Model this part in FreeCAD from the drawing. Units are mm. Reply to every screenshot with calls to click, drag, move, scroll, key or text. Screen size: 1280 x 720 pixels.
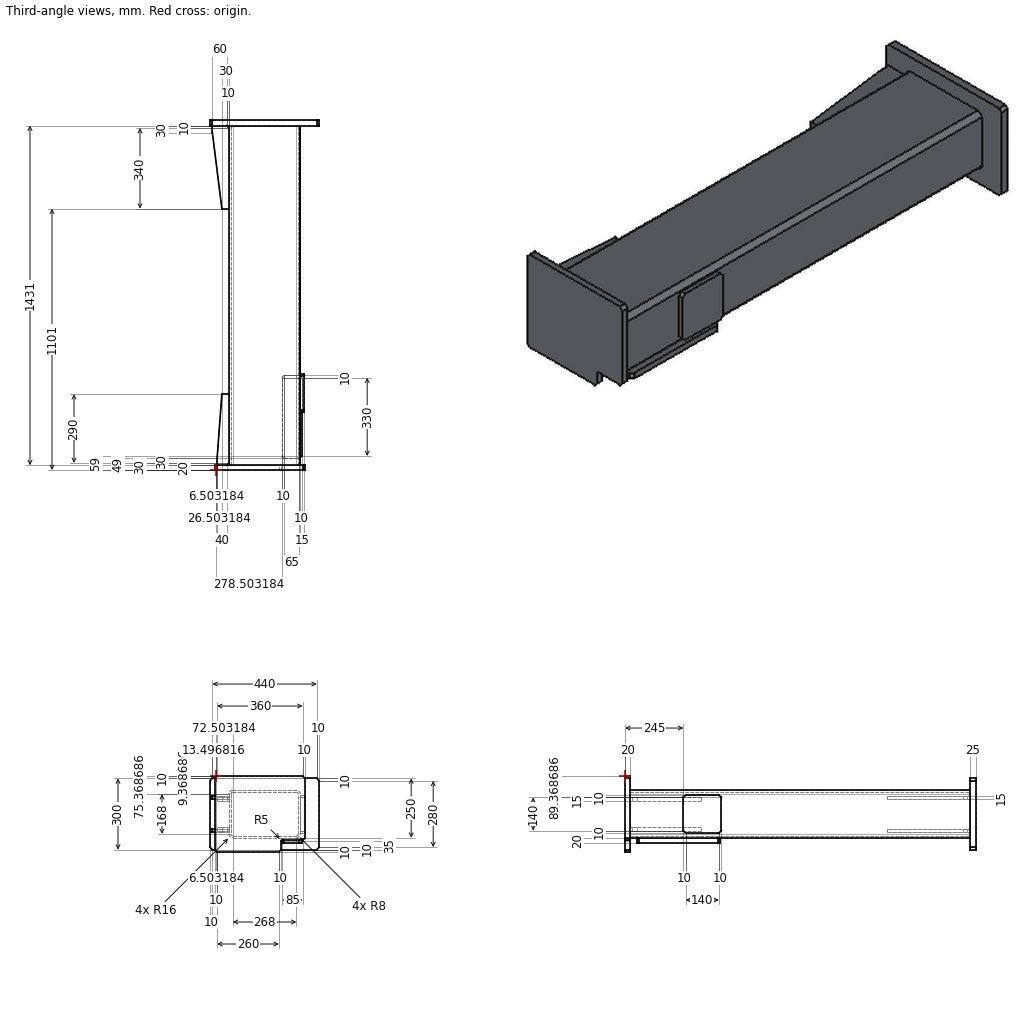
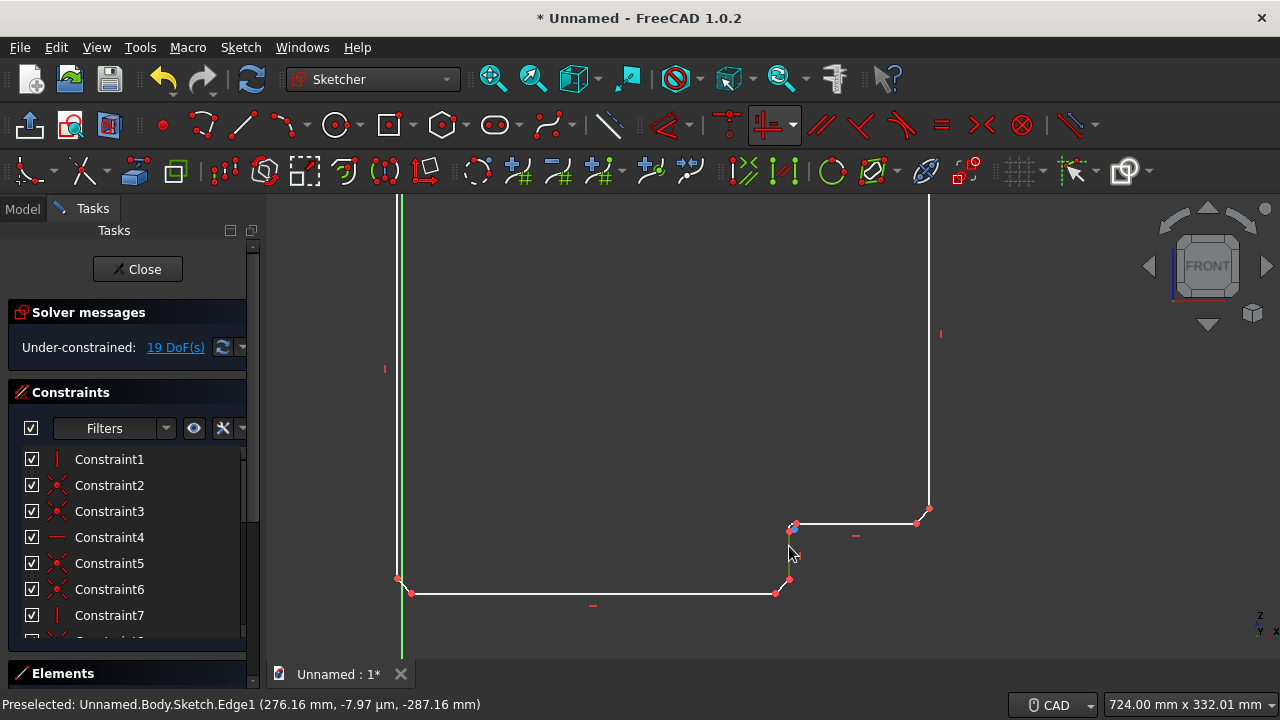
scroll(790, 525, up, 5)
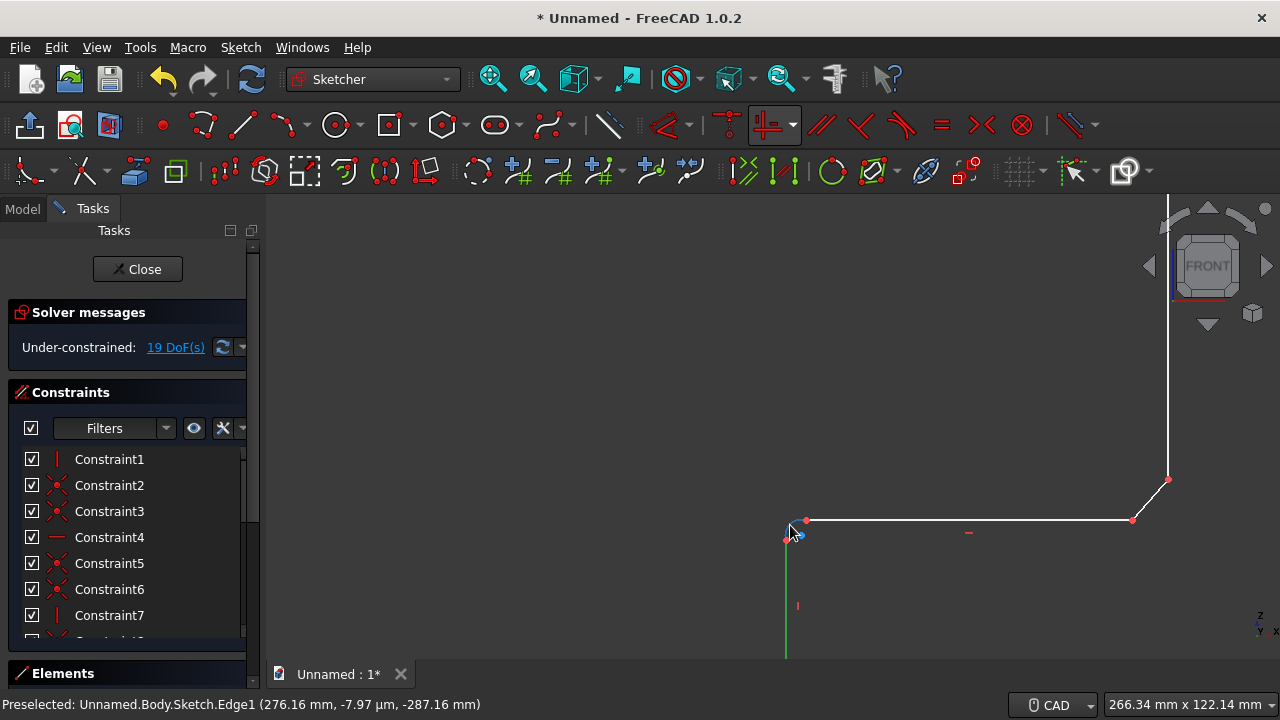
click(790, 524)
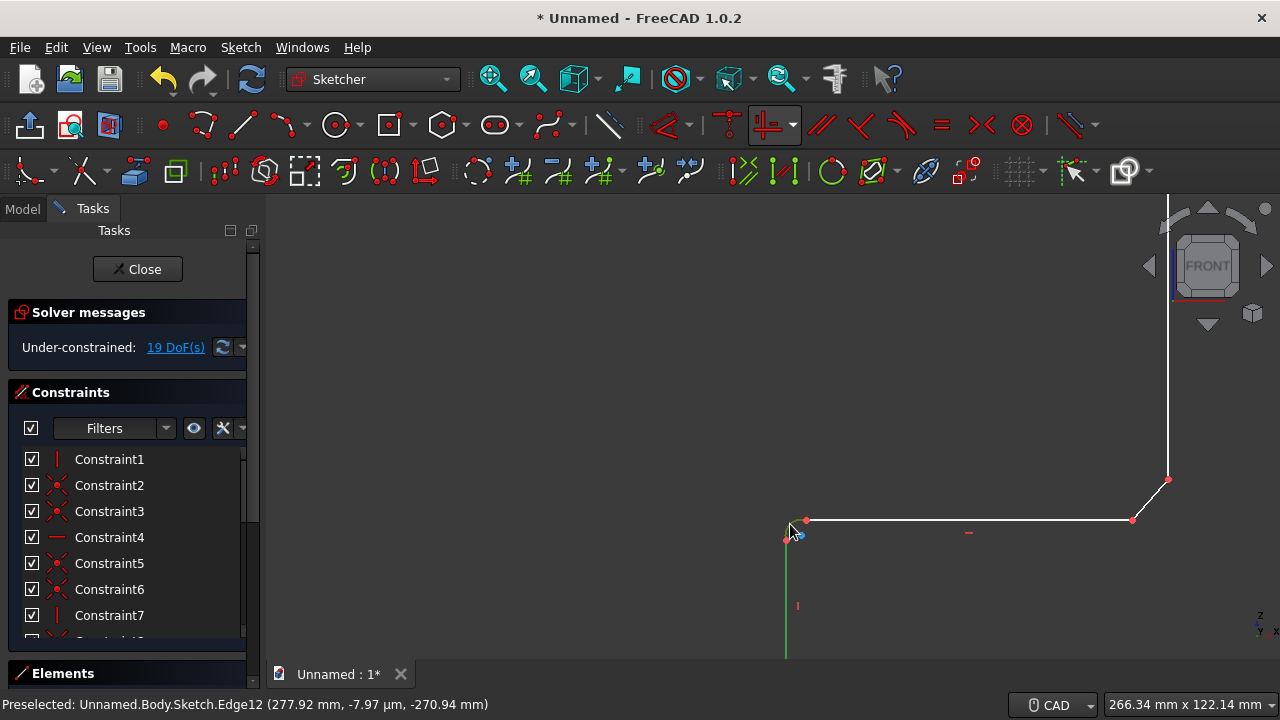
click(902, 126)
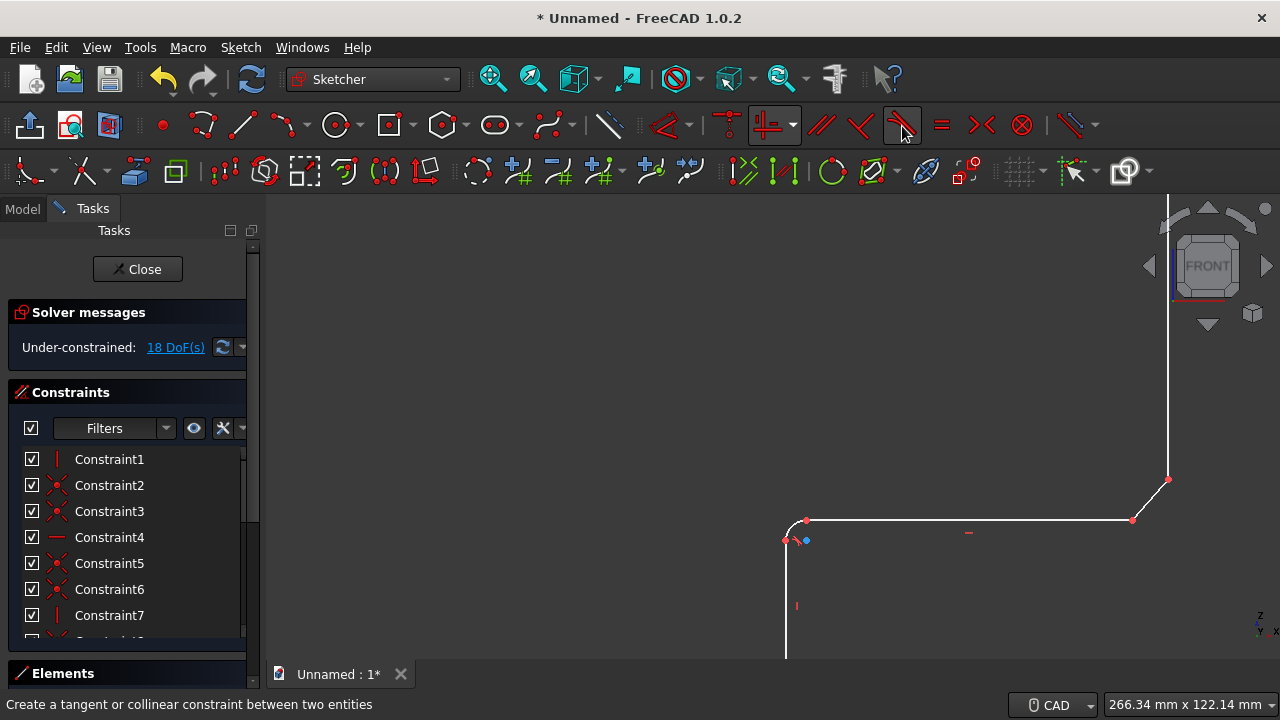
scroll(789, 534, down, 7)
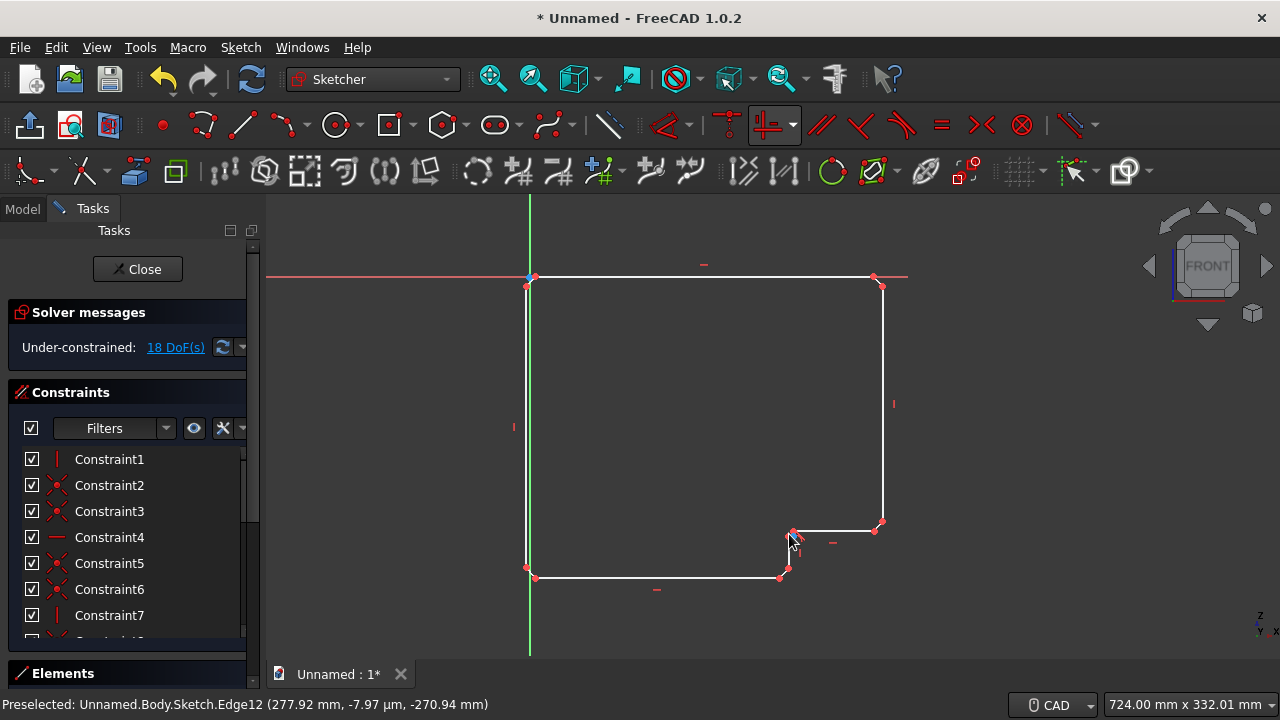
click(850, 531)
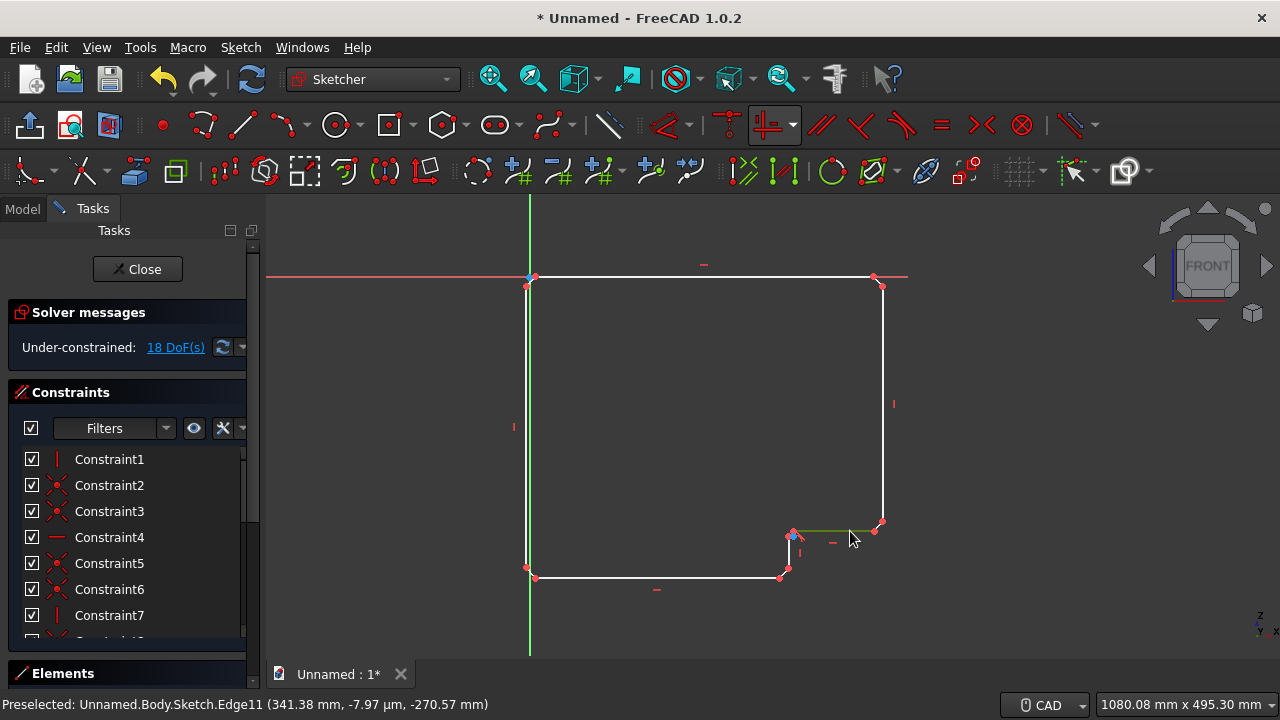
scroll(790, 533, up, 7)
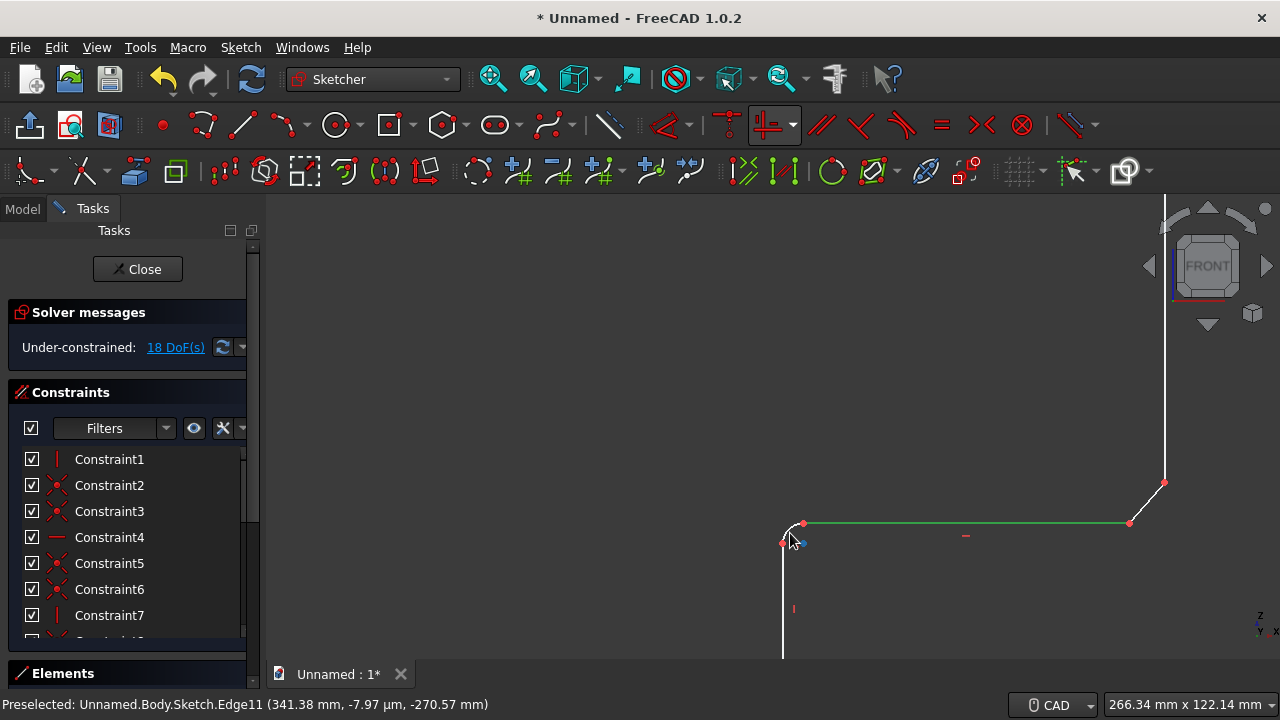
click(789, 529)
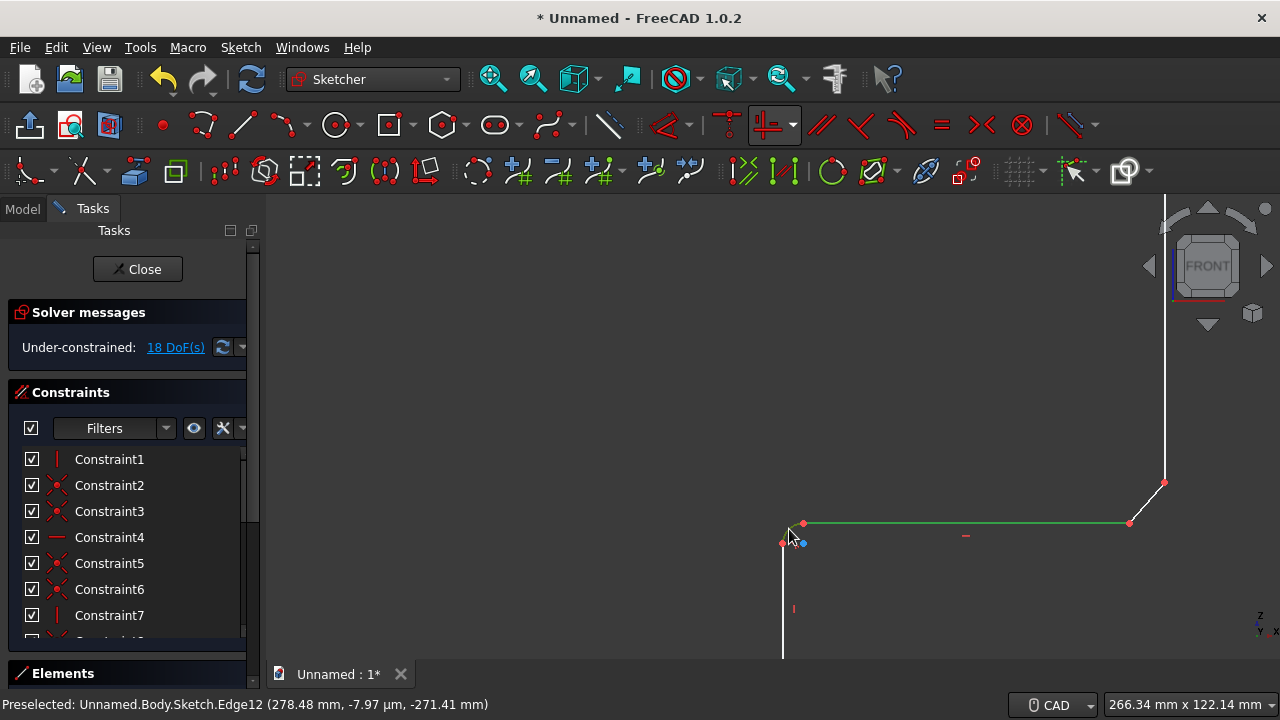
click(902, 126)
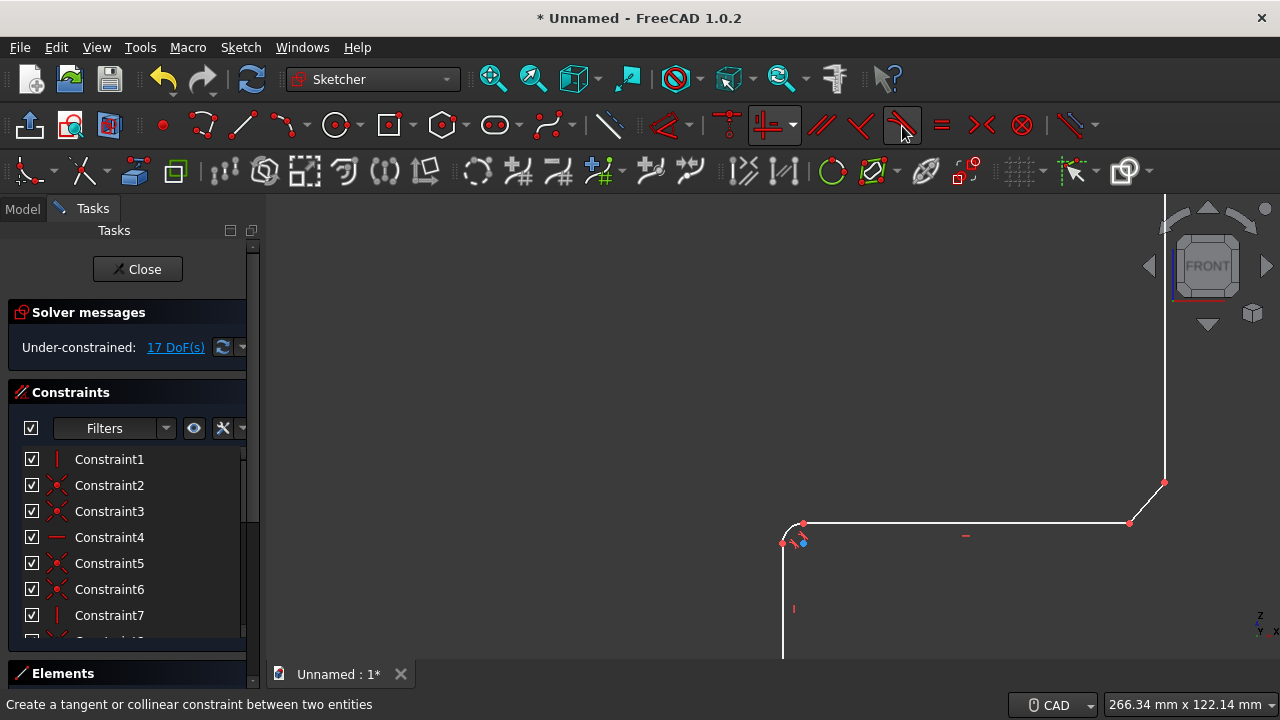
click(664, 126)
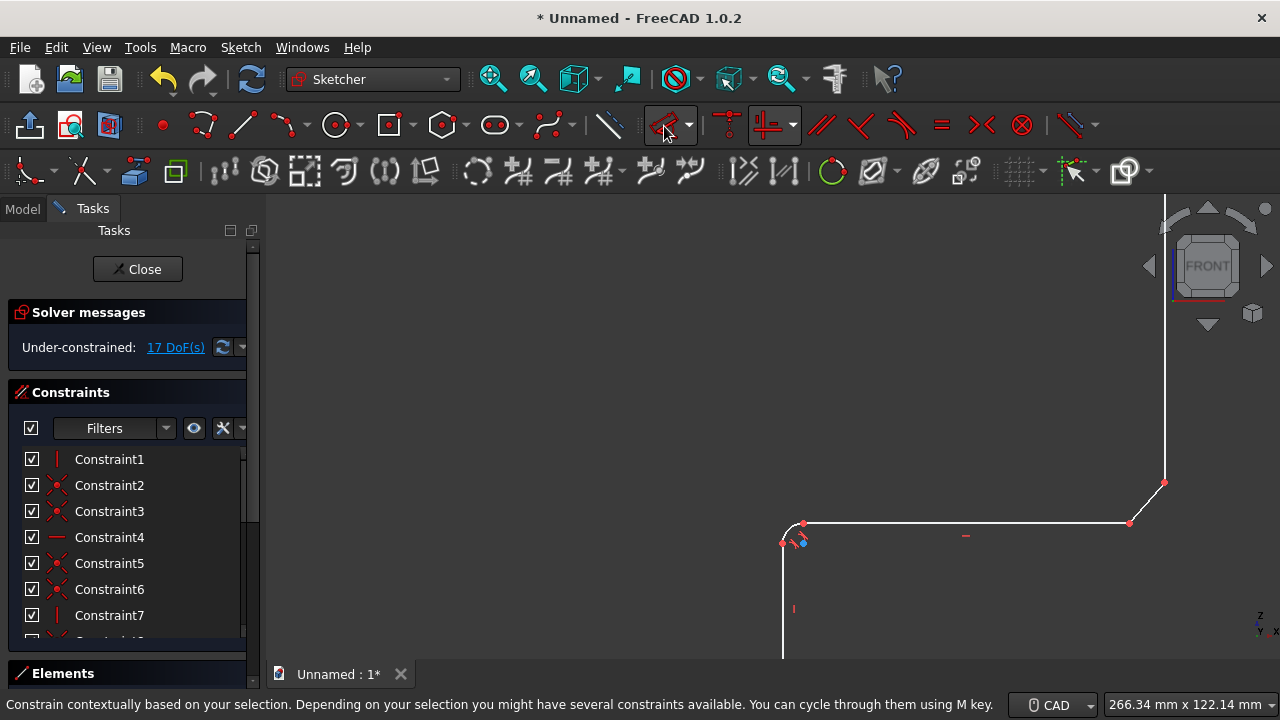
scroll(794, 526, up, 4)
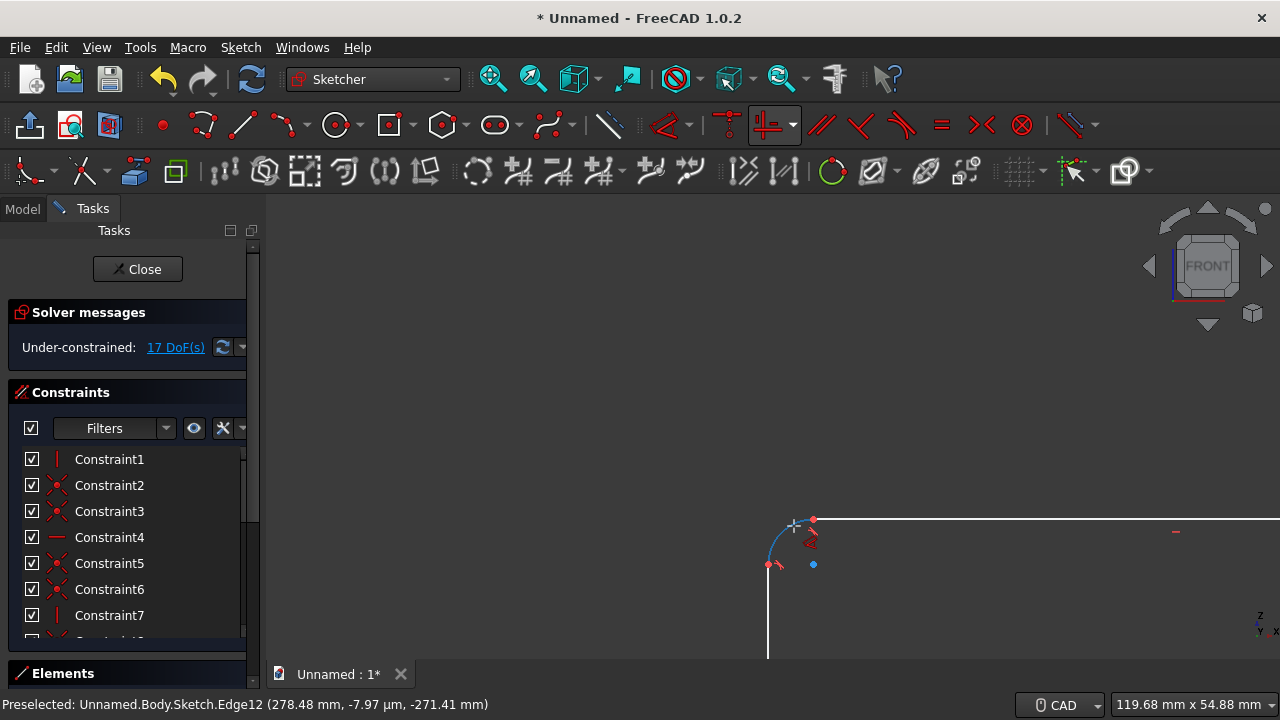
click(793, 524)
click(779, 495)